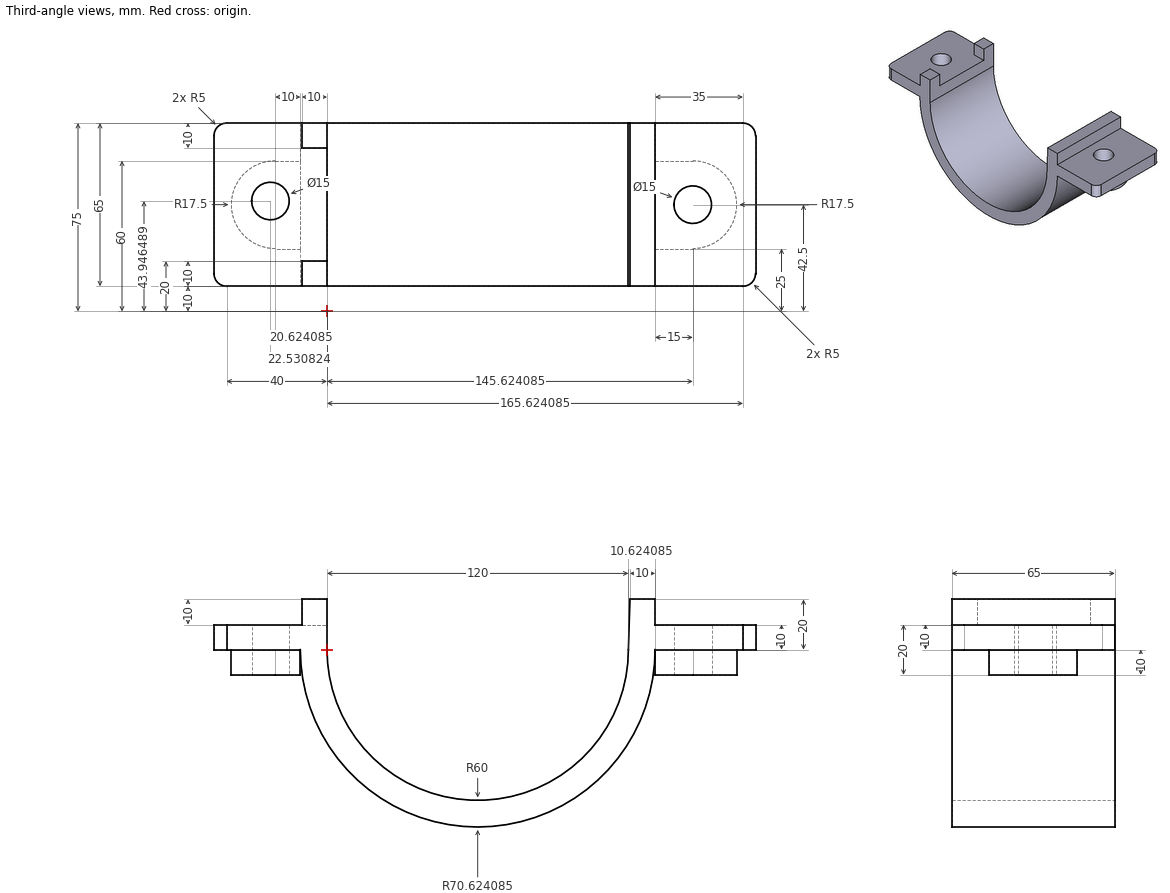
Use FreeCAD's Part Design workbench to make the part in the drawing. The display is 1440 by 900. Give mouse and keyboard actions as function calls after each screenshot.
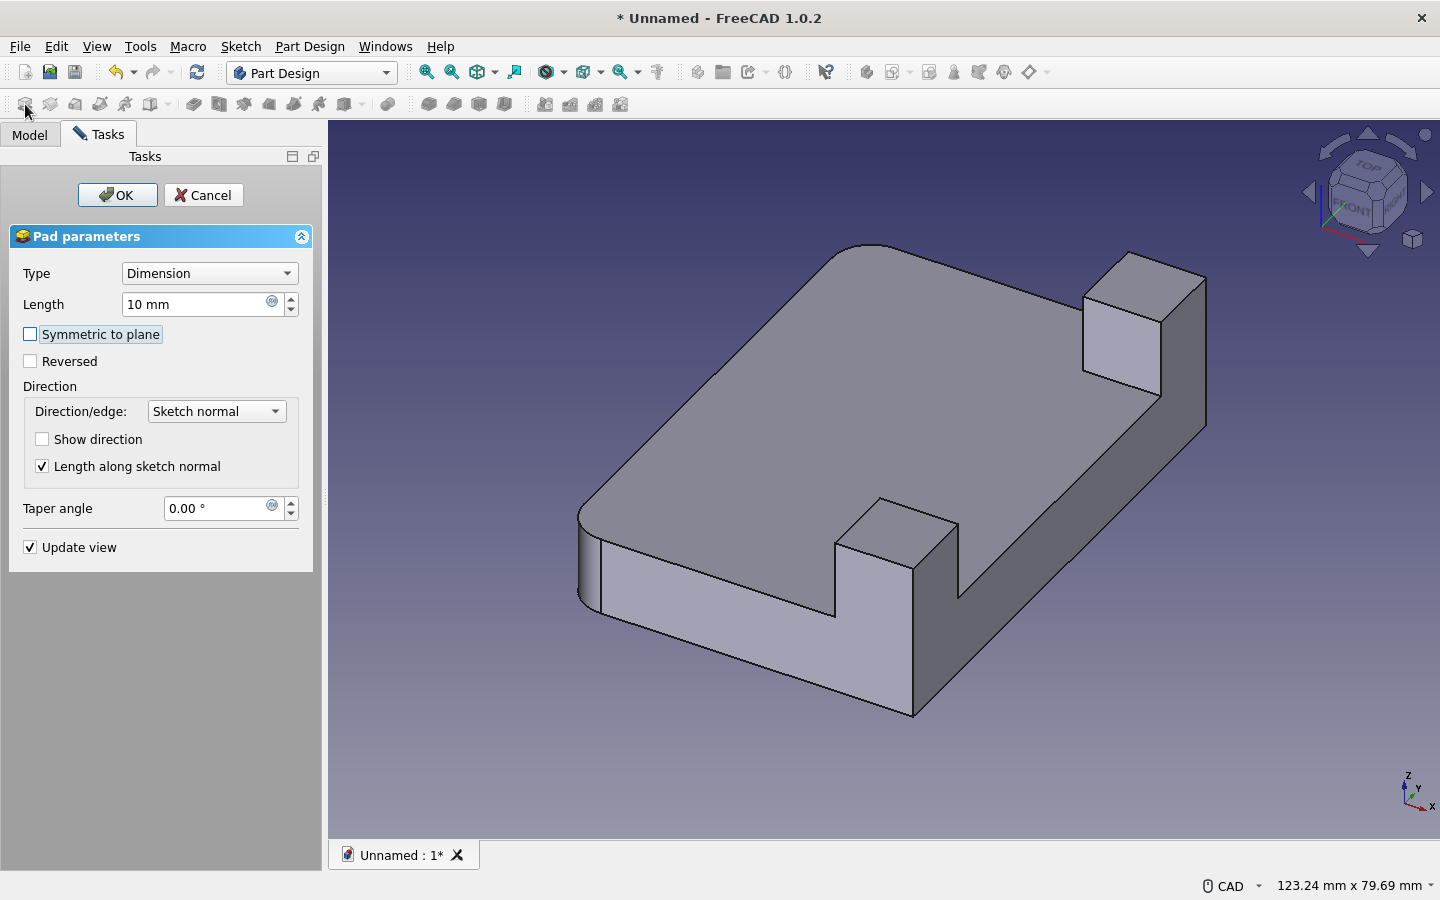
click(118, 195)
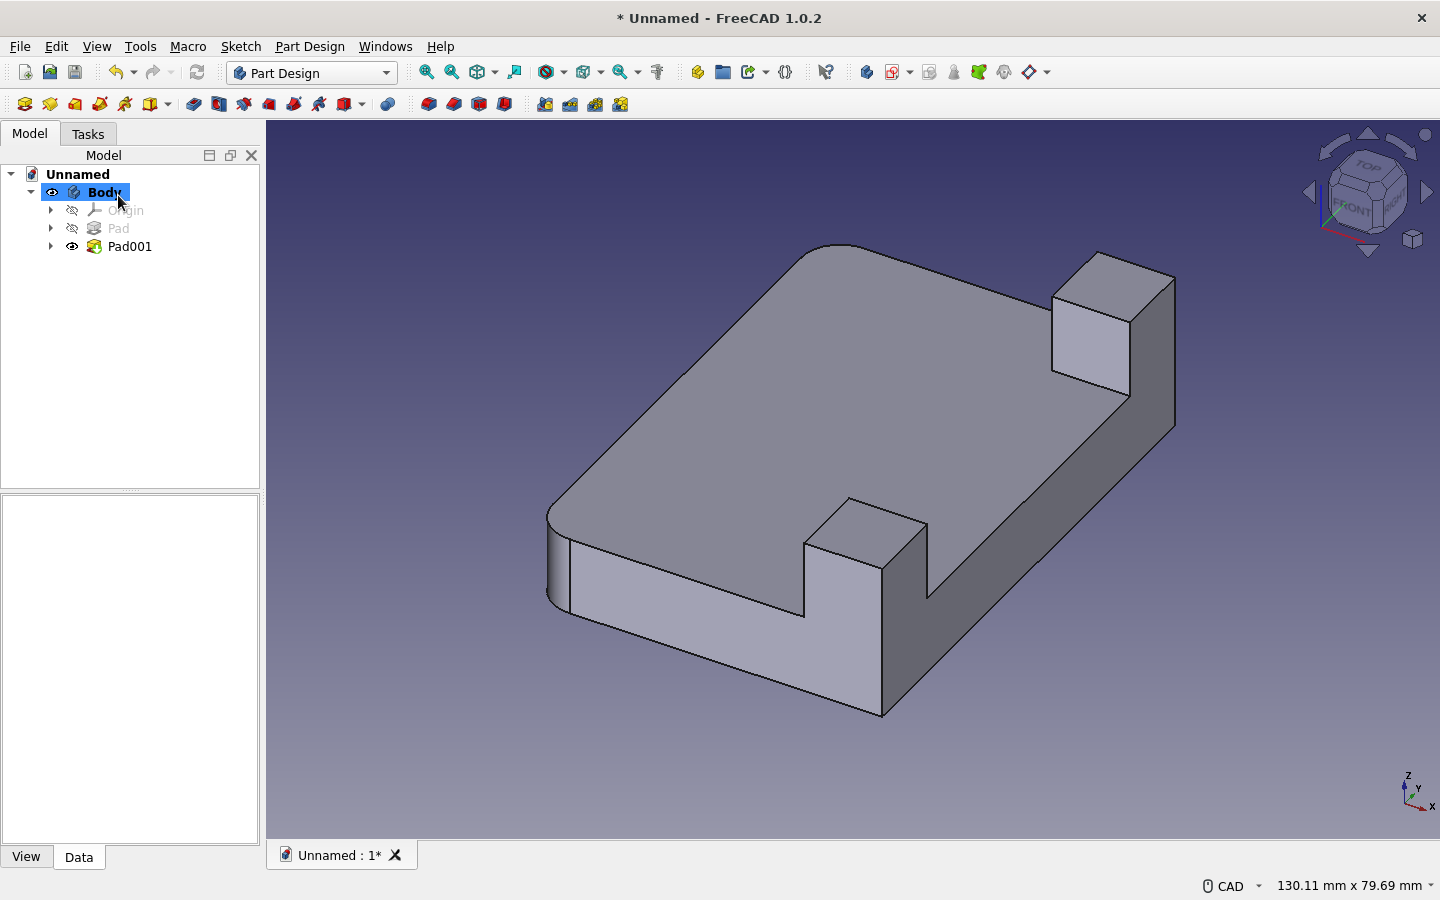
key(4)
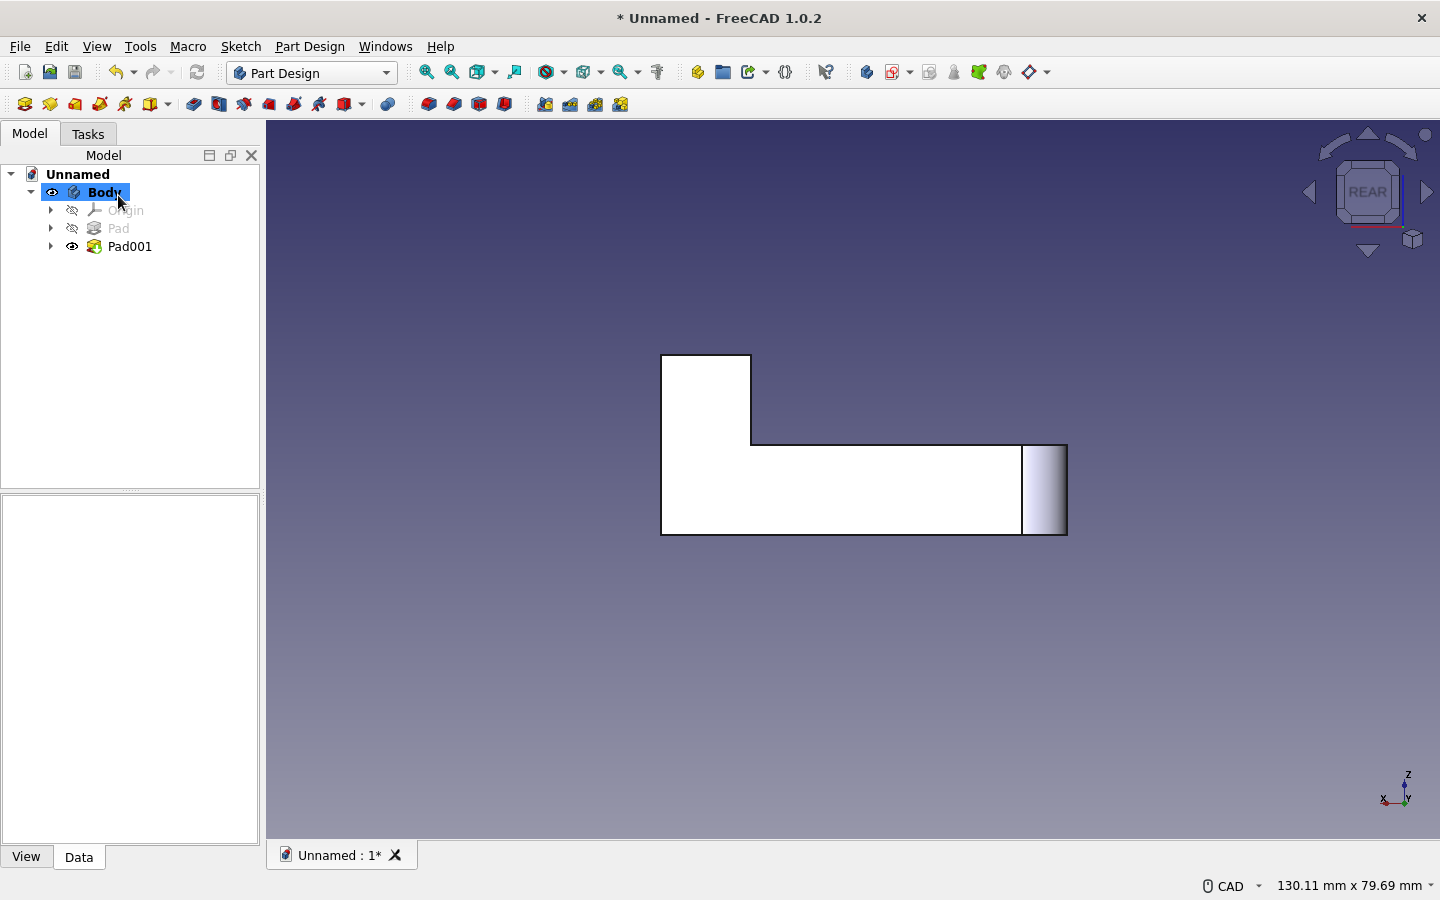
key(v)
key(f)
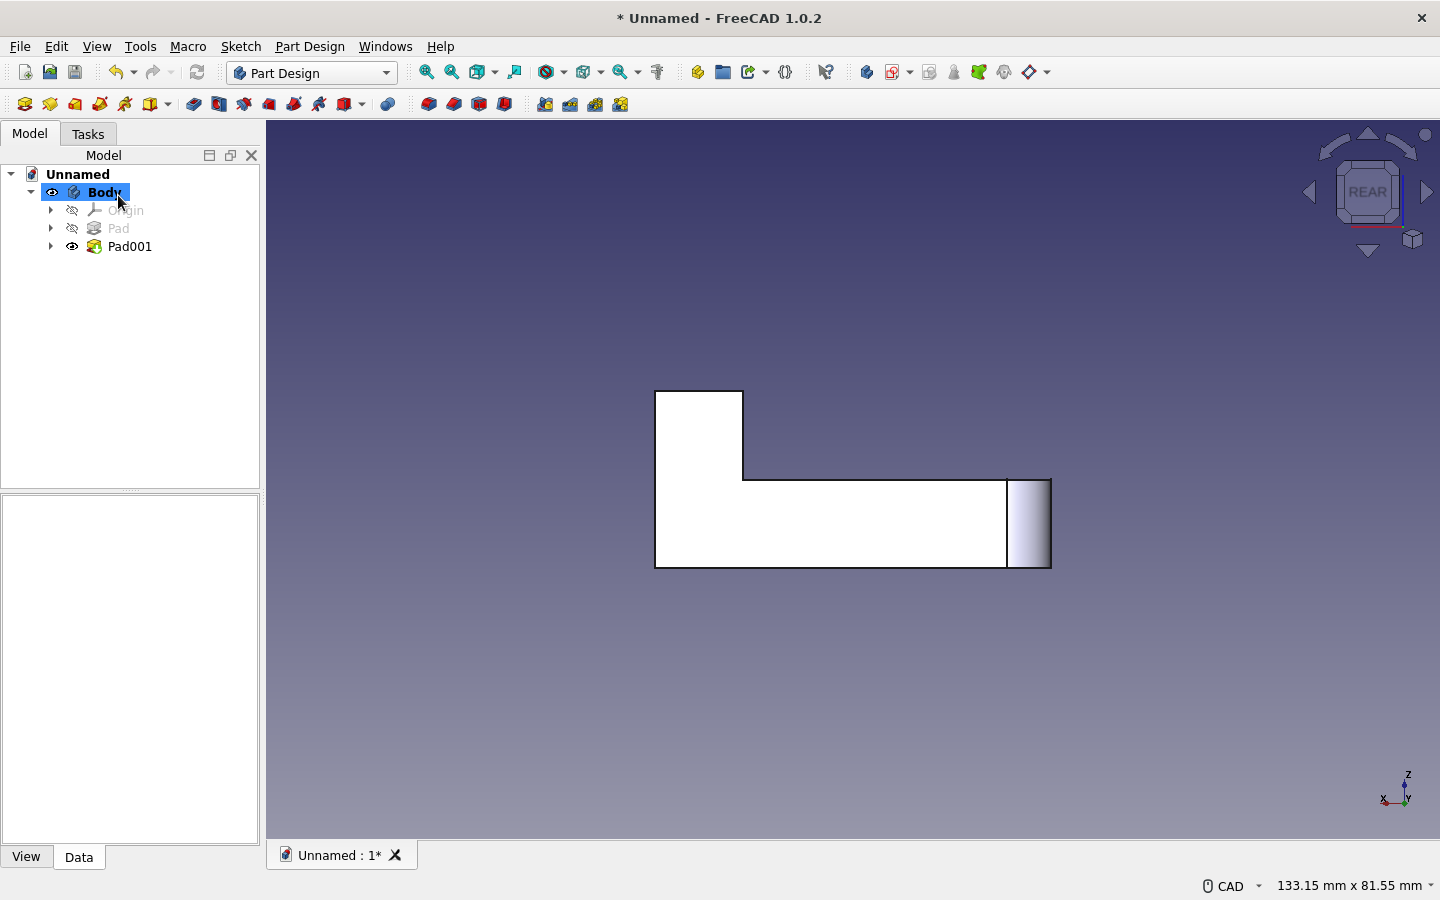
click(730, 529)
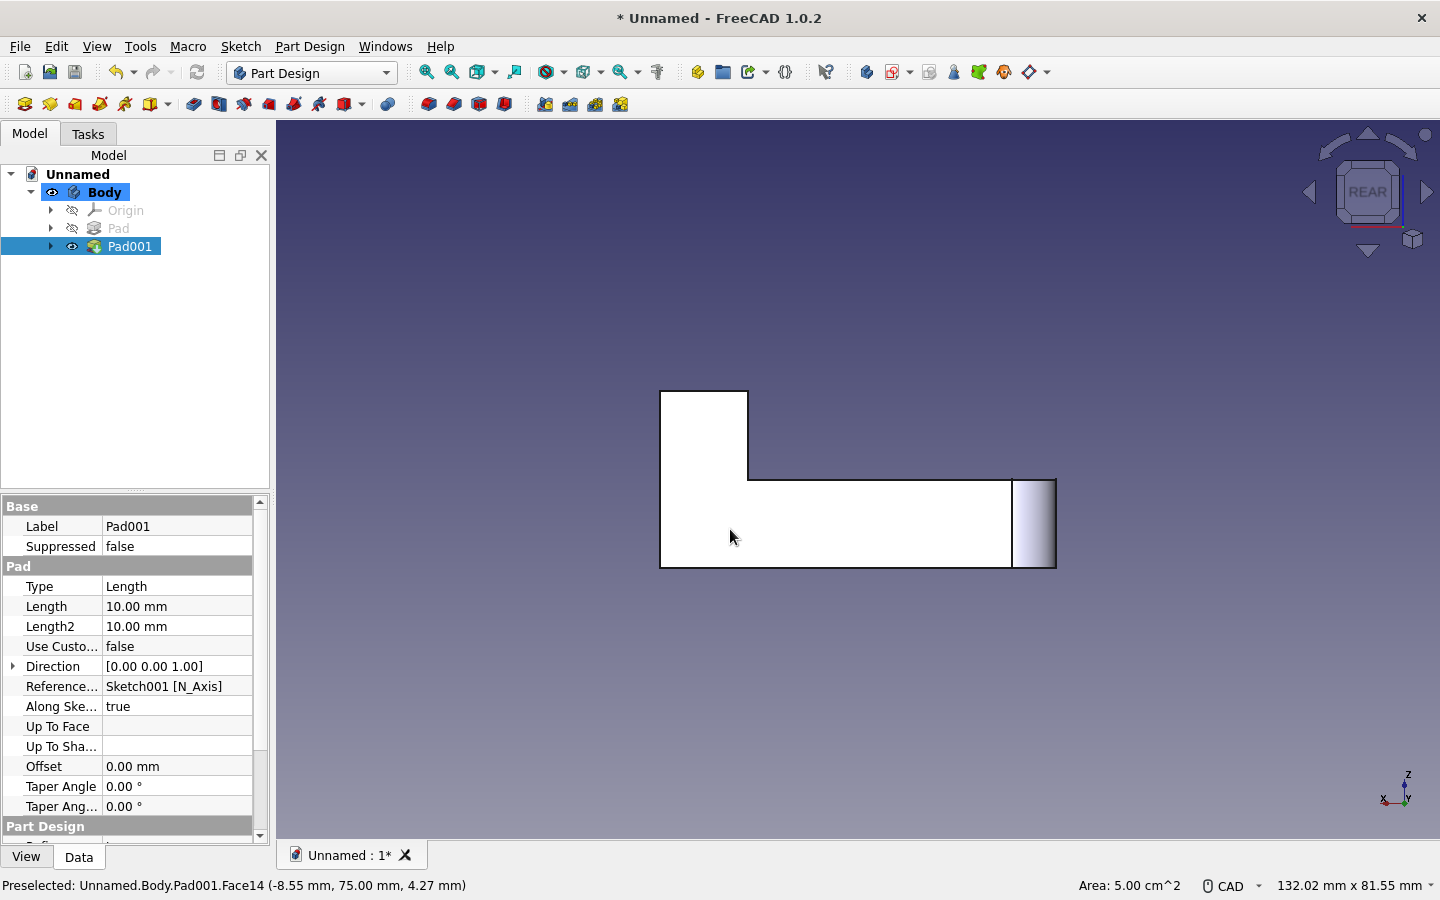
click(892, 72)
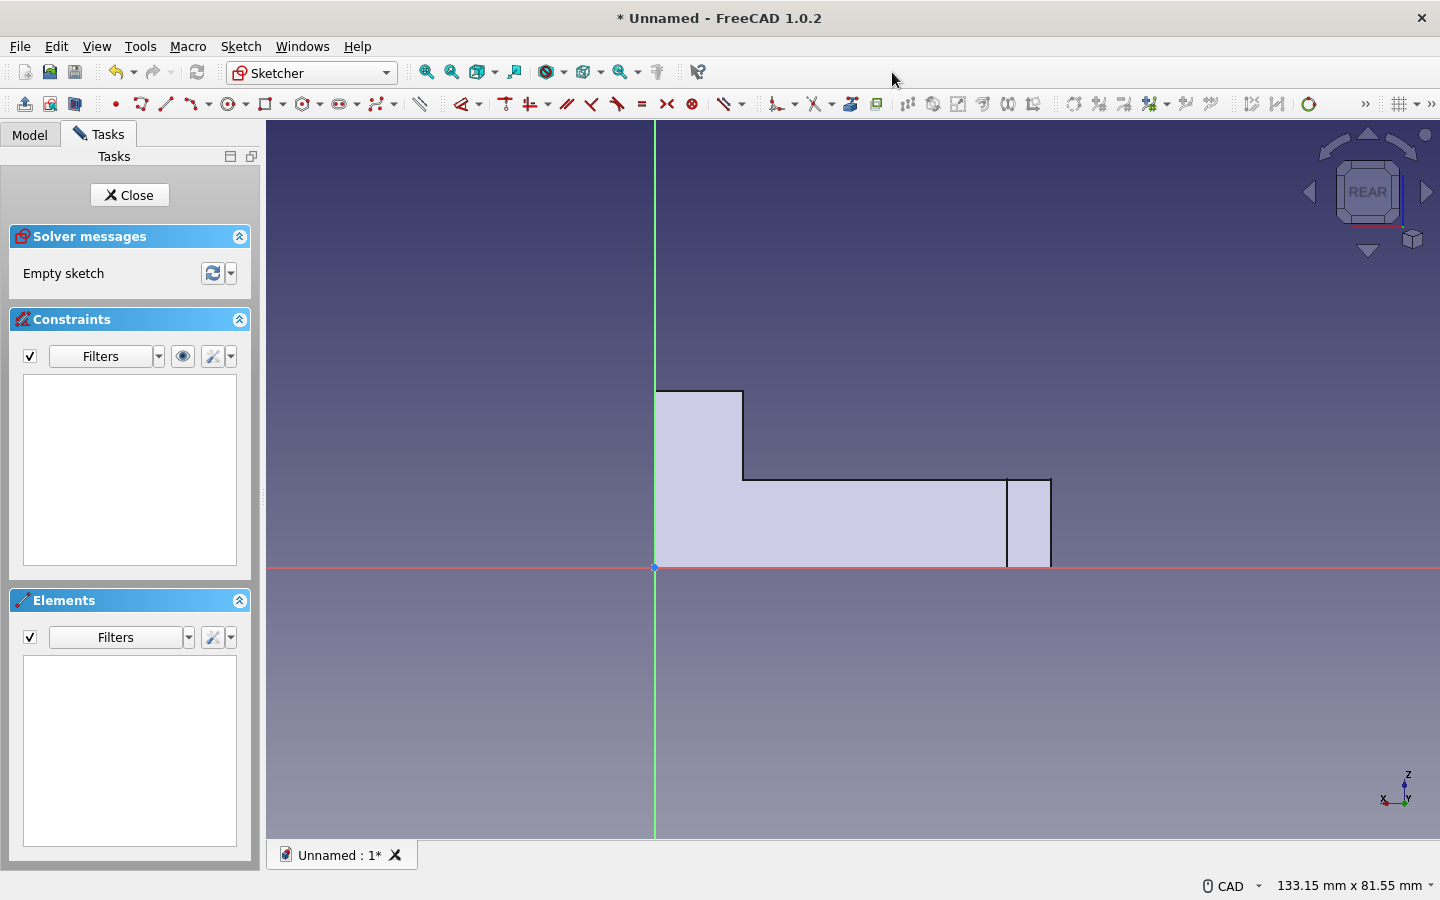
scroll(1275, 154, down, 4)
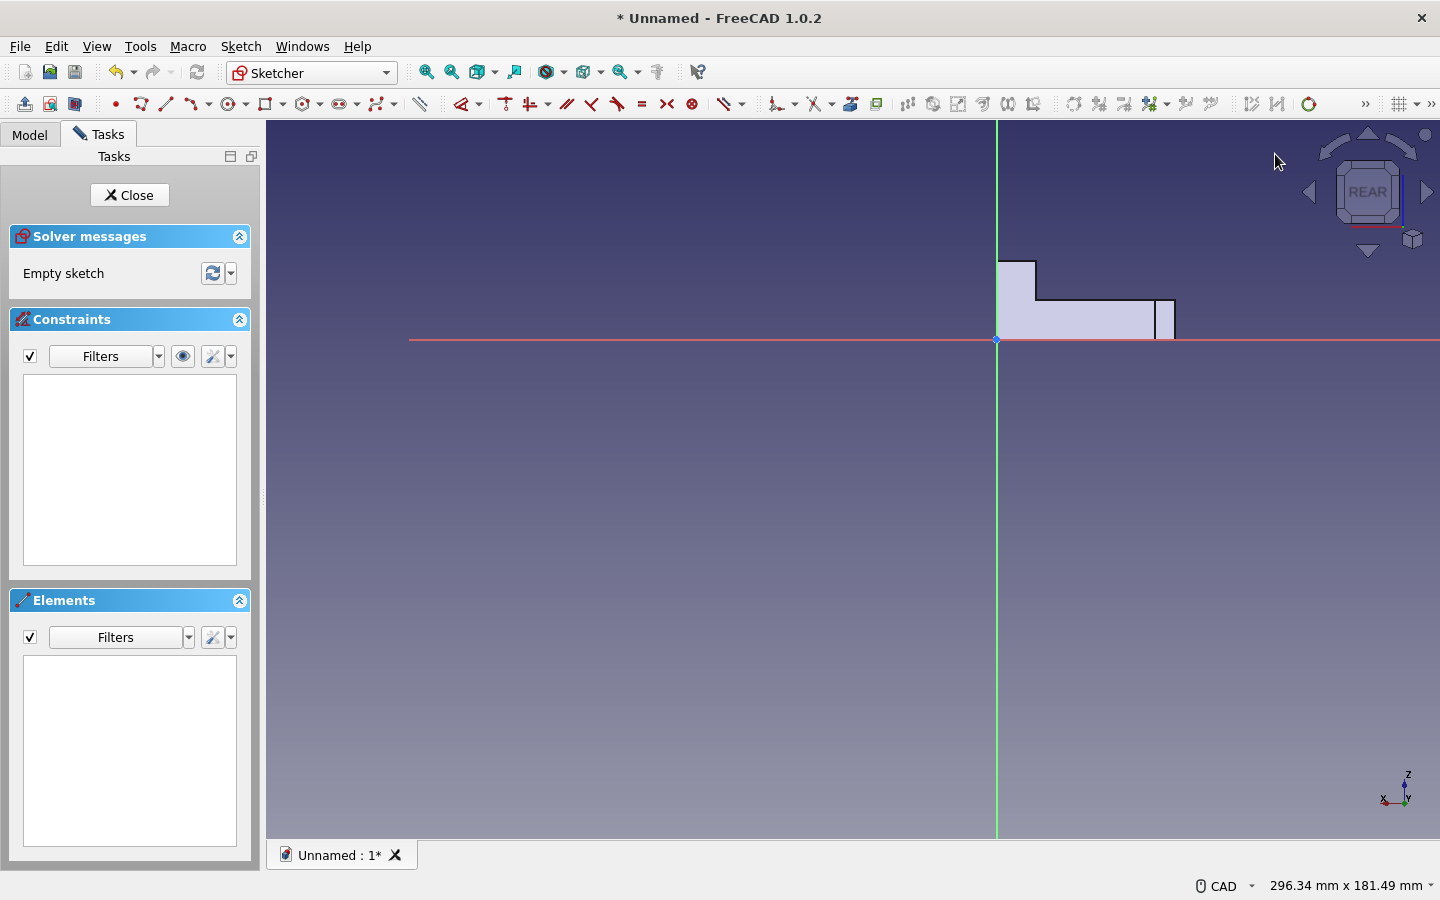
key(g)
key(l)